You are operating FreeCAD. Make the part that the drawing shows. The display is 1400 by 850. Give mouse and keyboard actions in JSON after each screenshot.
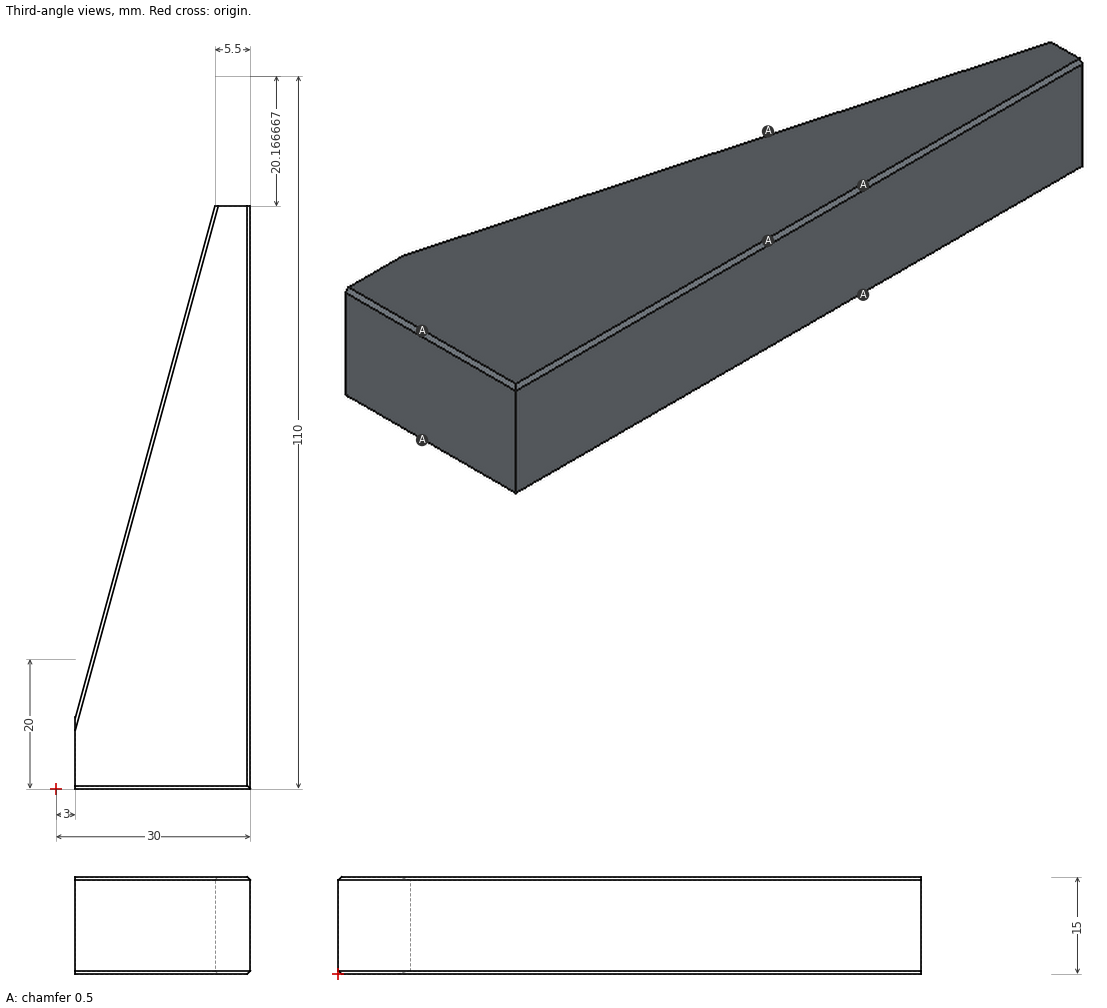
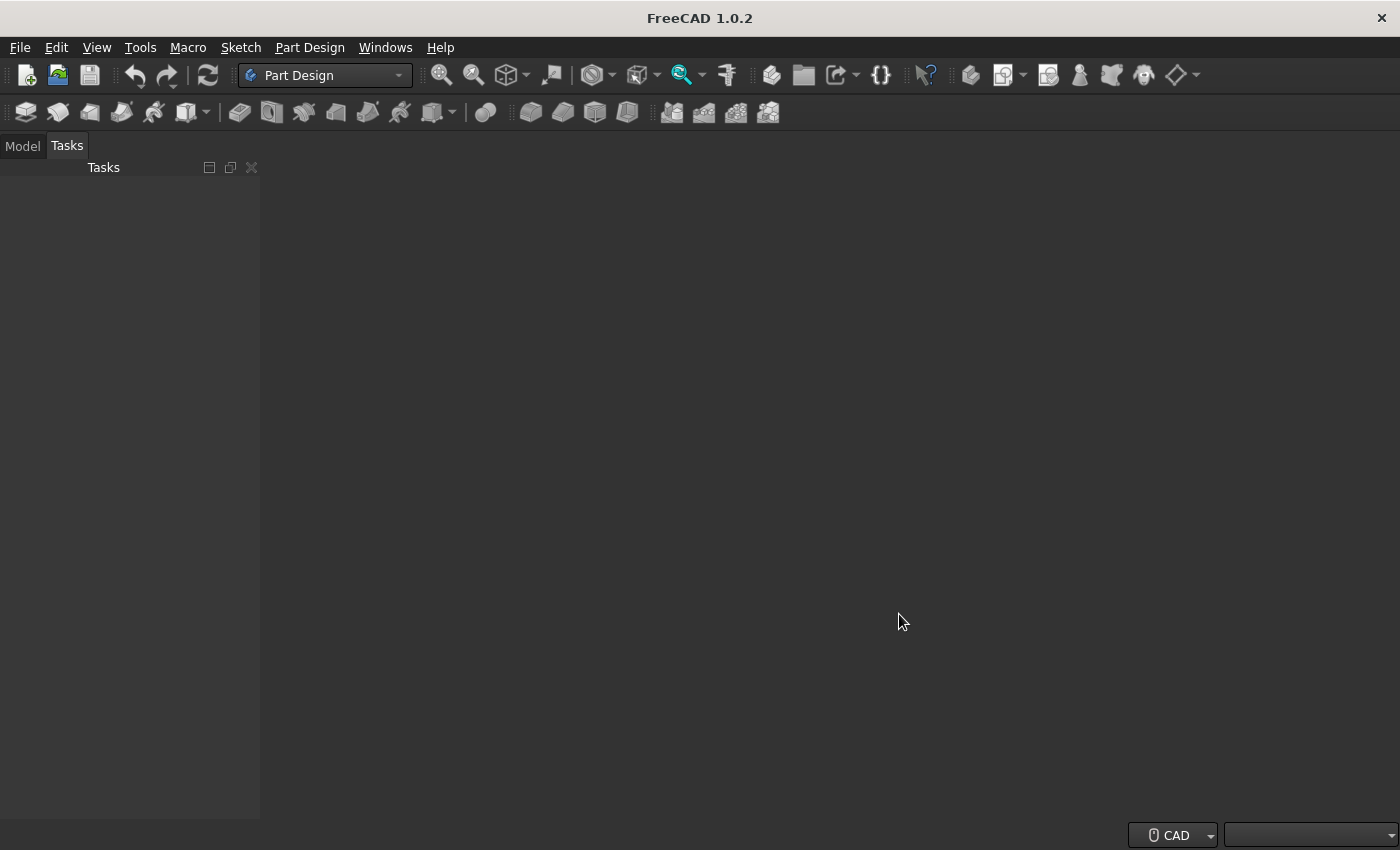
{"action": "left_click", "coordinate": [26, 76]}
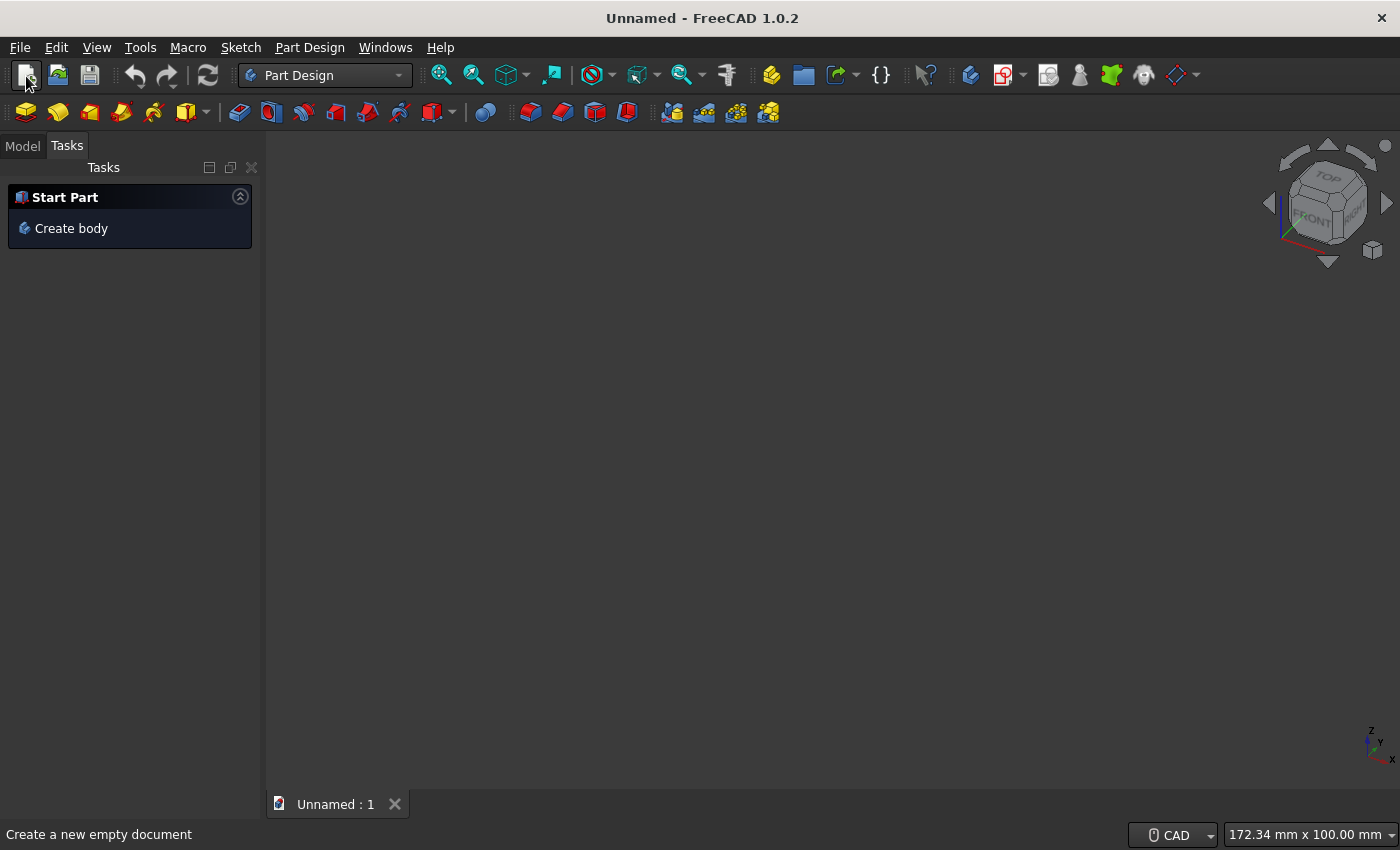
{"action": "left_click", "coordinate": [1004, 76]}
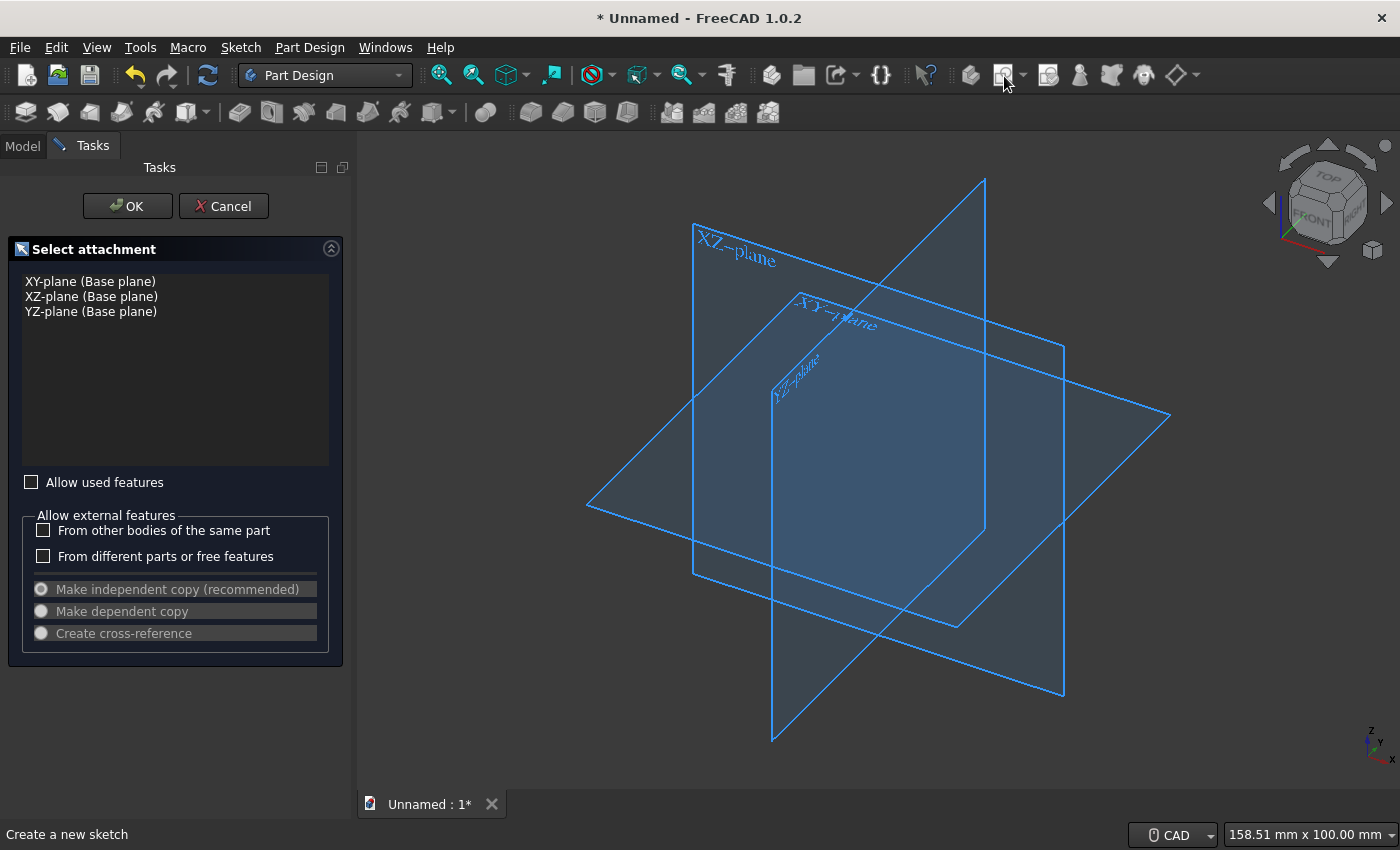
{"action": "left_click", "coordinate": [82, 282]}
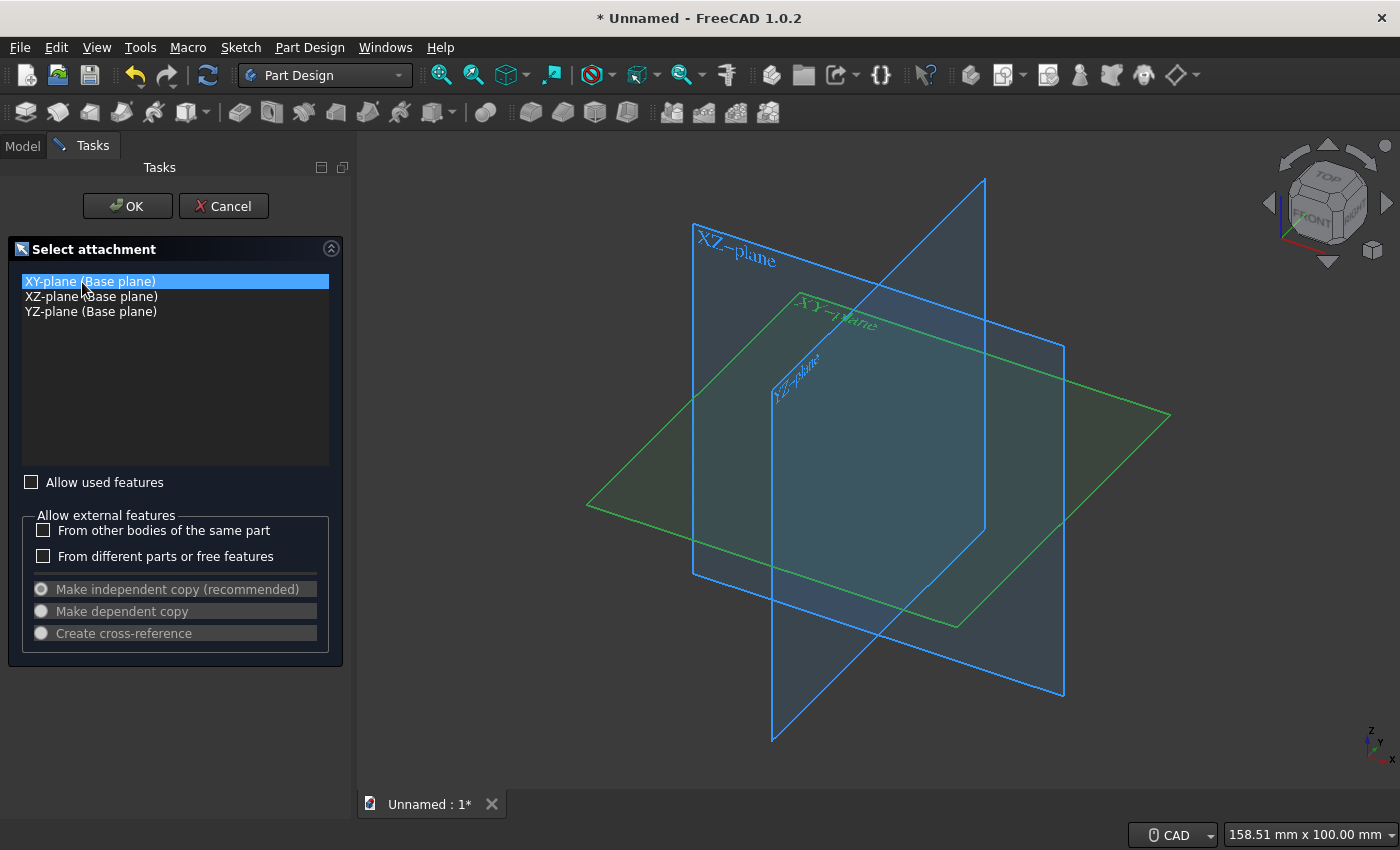
{"action": "left_click", "coordinate": [128, 206]}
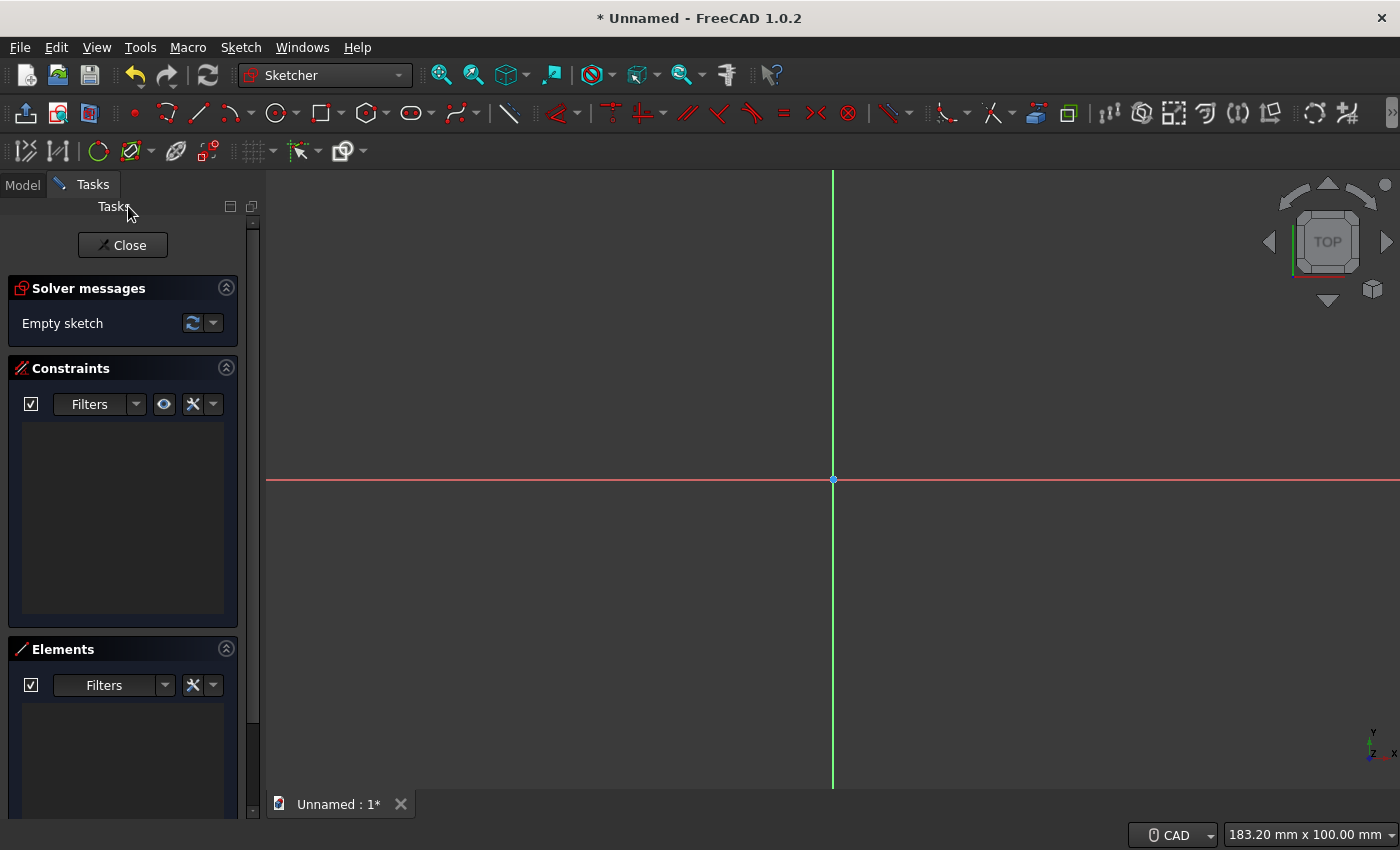
{"action": "scroll", "coordinate": [568, 761], "scroll_direction": "down", "scroll_amount": 3}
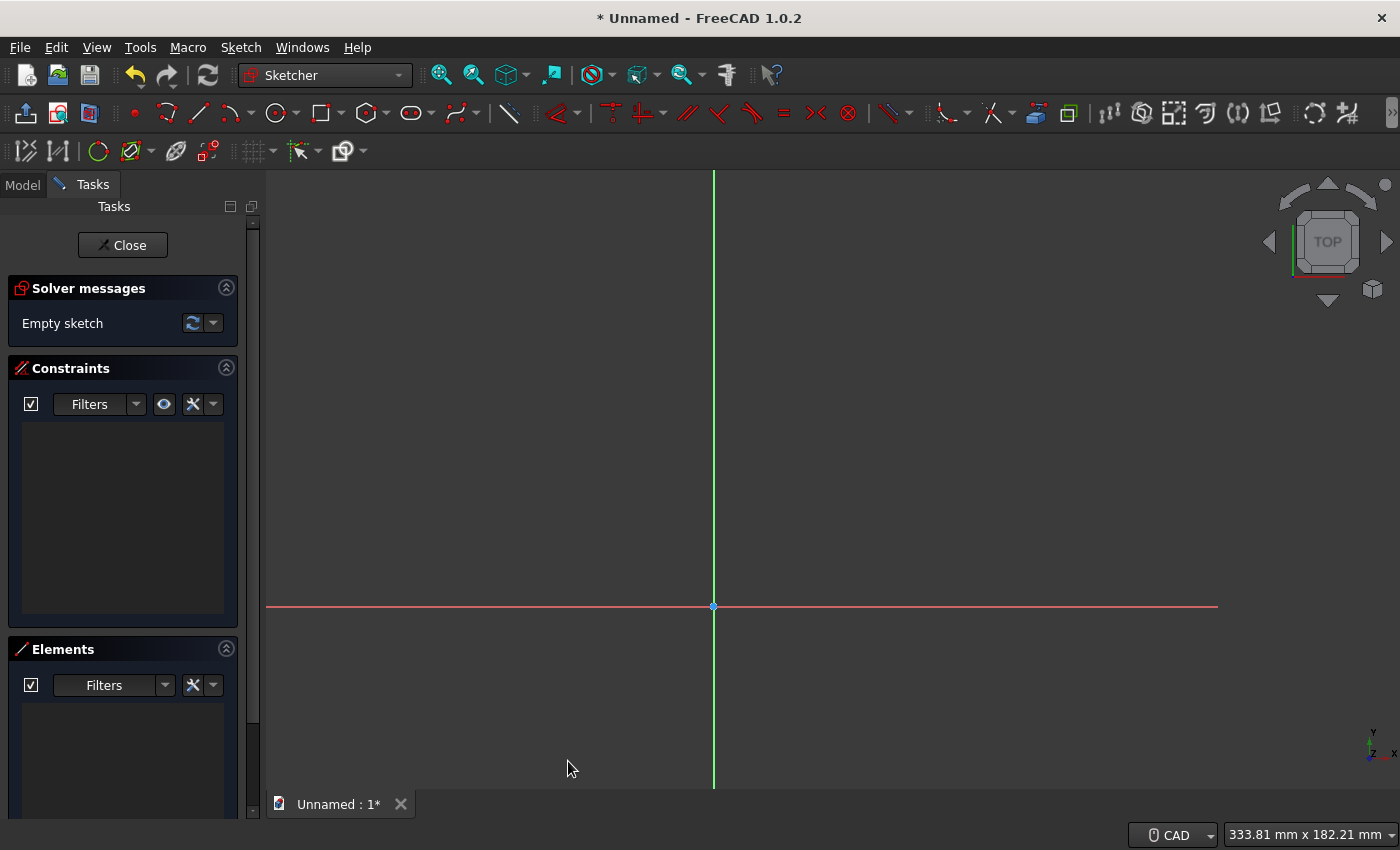
{"action": "left_click", "coordinate": [168, 114]}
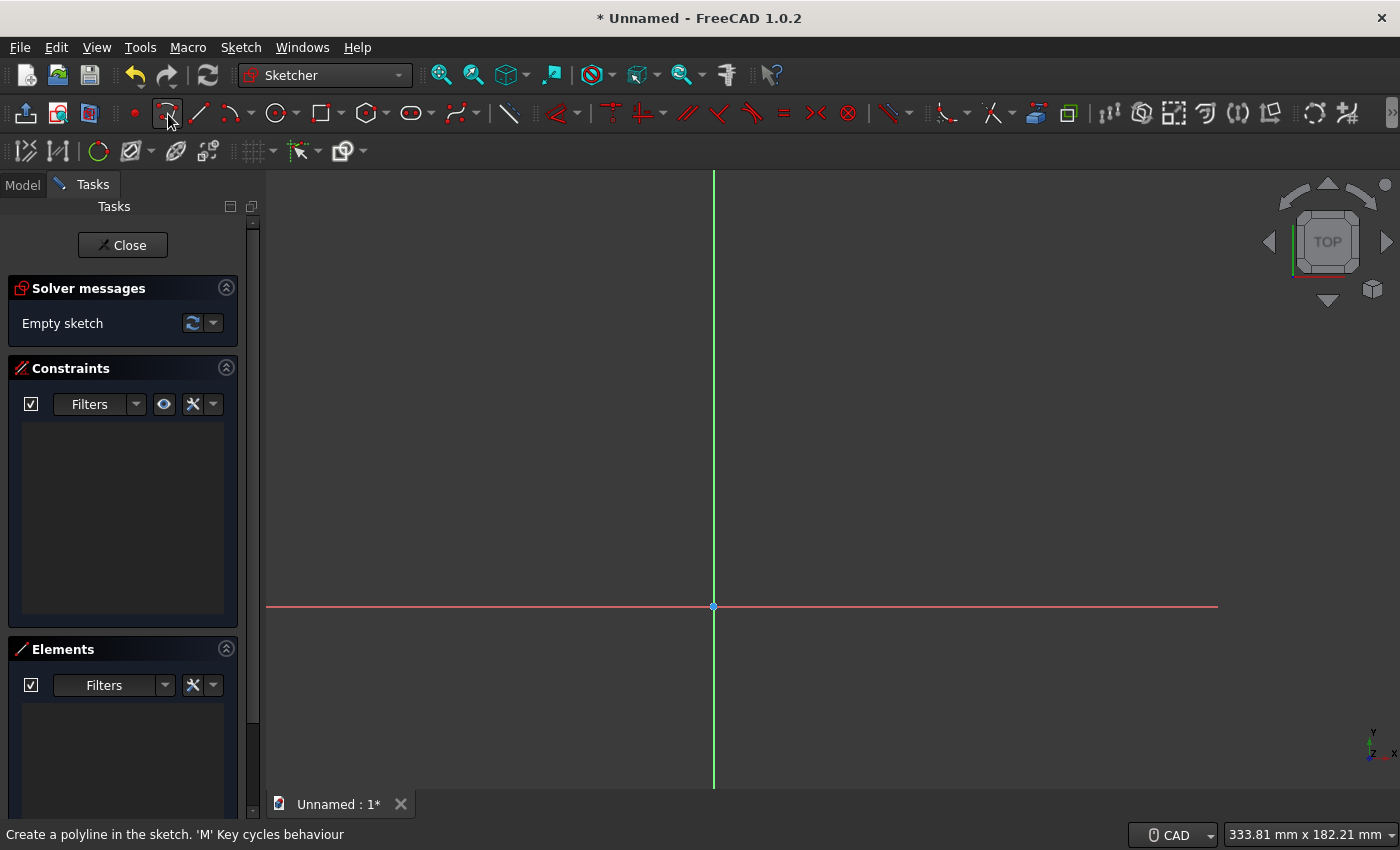
{"action": "left_click", "coordinate": [714, 607]}
{"action": "left_click", "coordinate": [815, 598]}
{"action": "left_click", "coordinate": [815, 233]}
{"action": "left_click", "coordinate": [714, 607]}
{"action": "key", "text": "Escape"}
{"action": "key", "text": "Escape"}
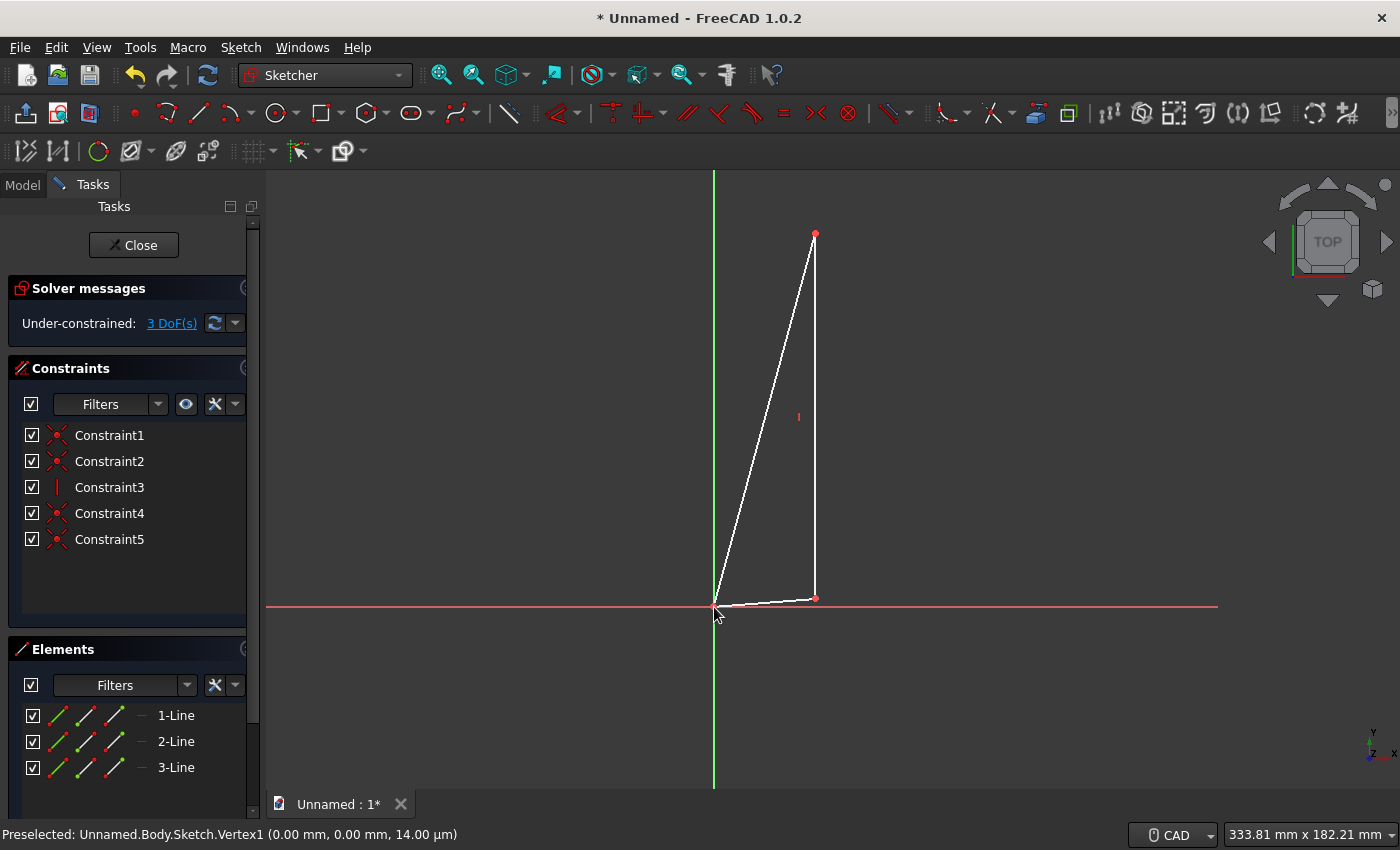
{"action": "left_click", "coordinate": [744, 605]}